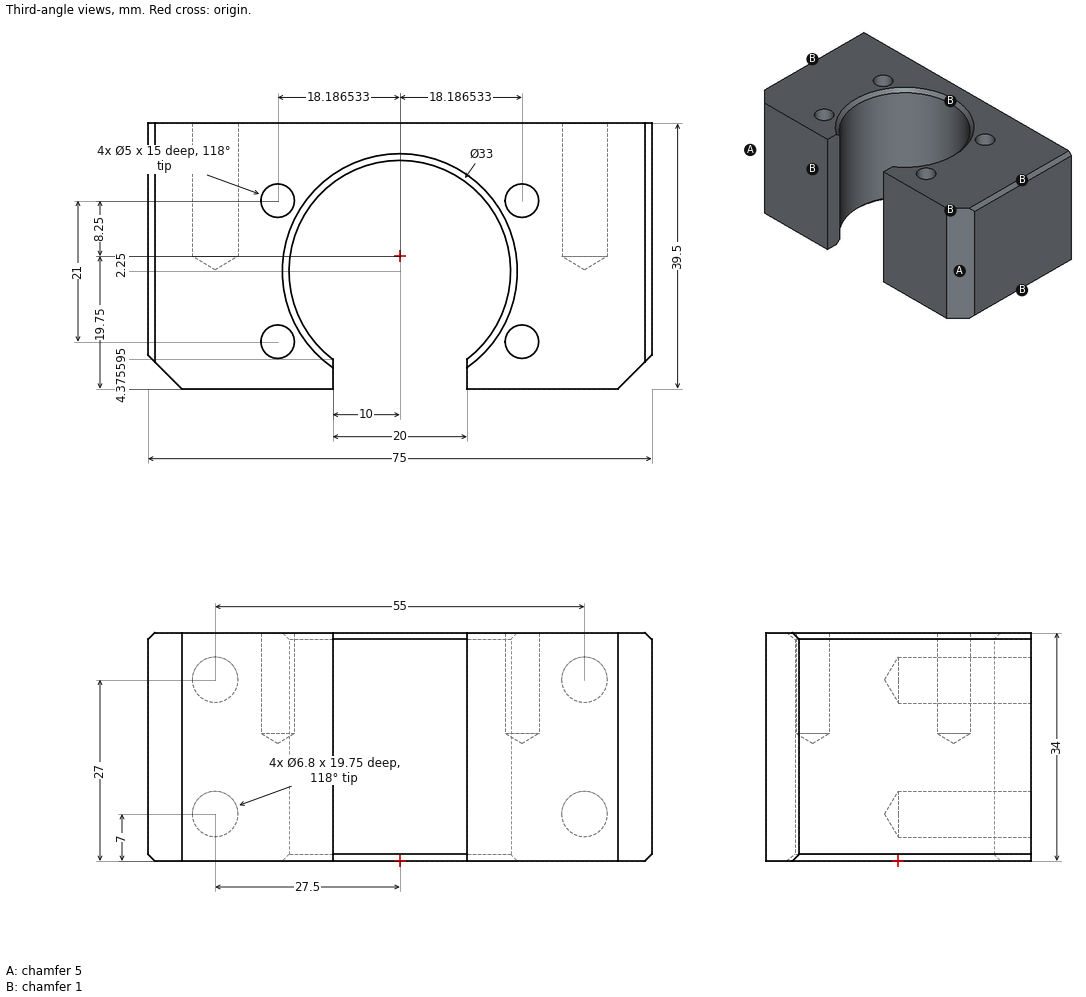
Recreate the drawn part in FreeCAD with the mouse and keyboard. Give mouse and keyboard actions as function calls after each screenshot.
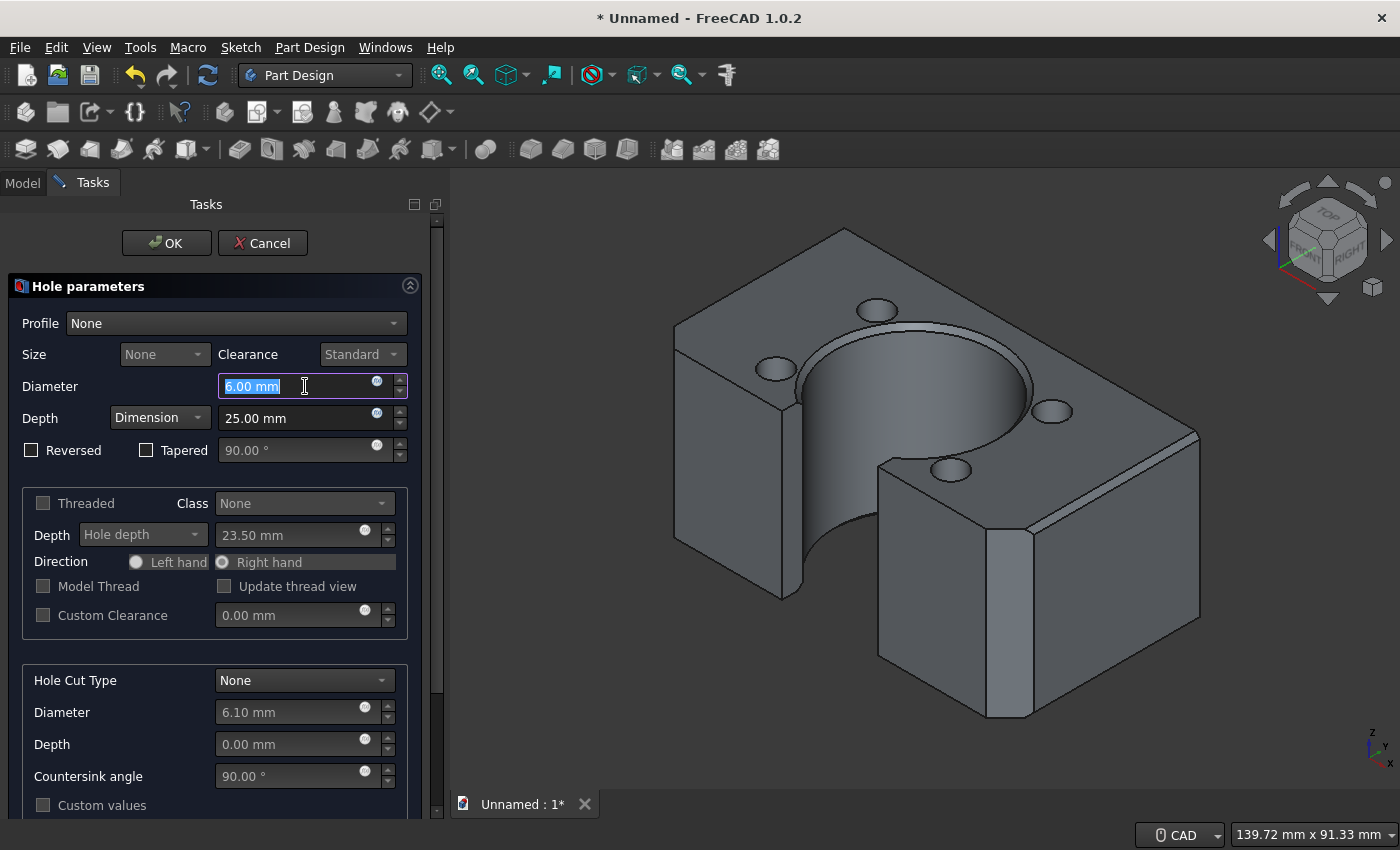
text(5)
key(Tab)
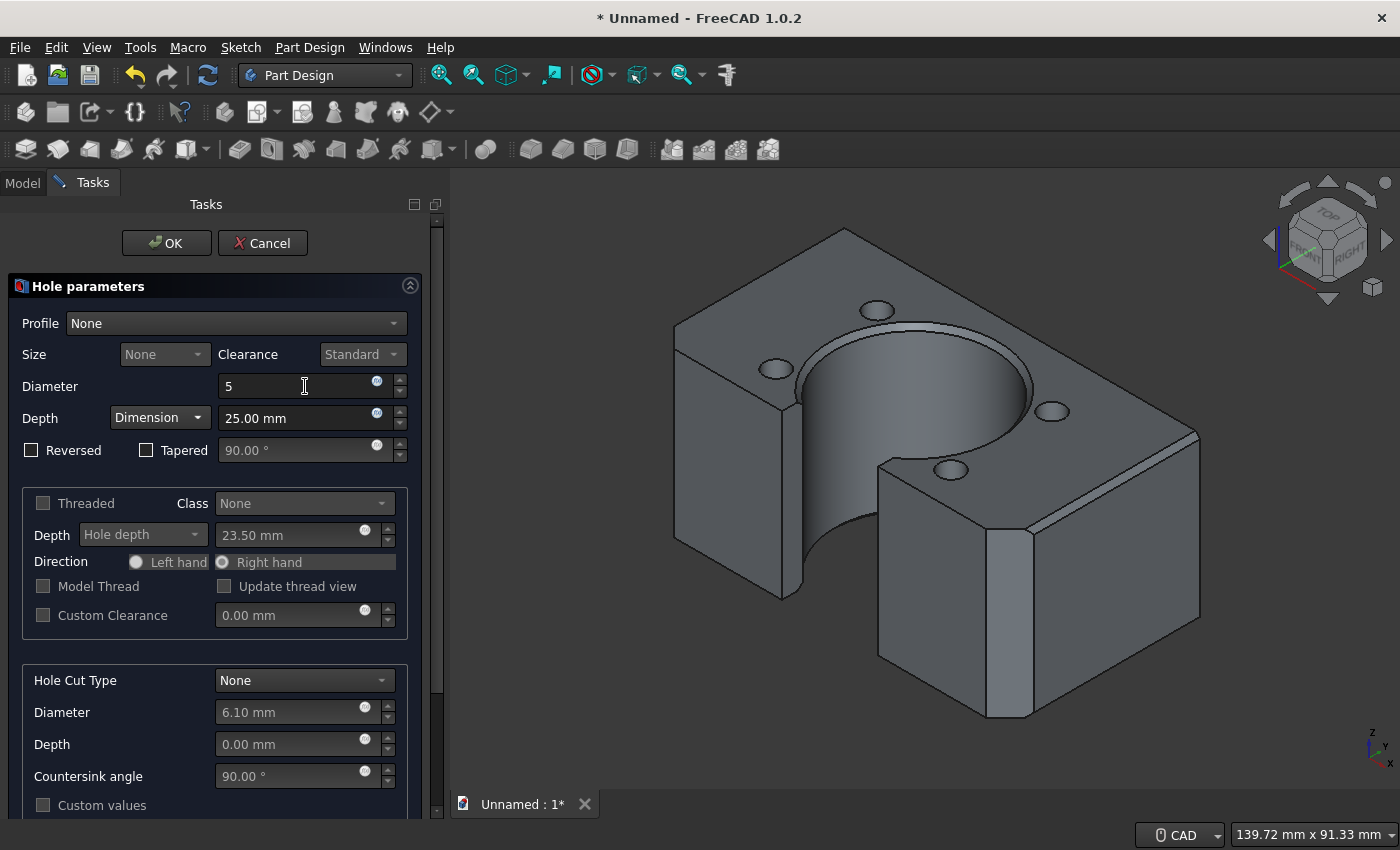
triple_click(305, 418)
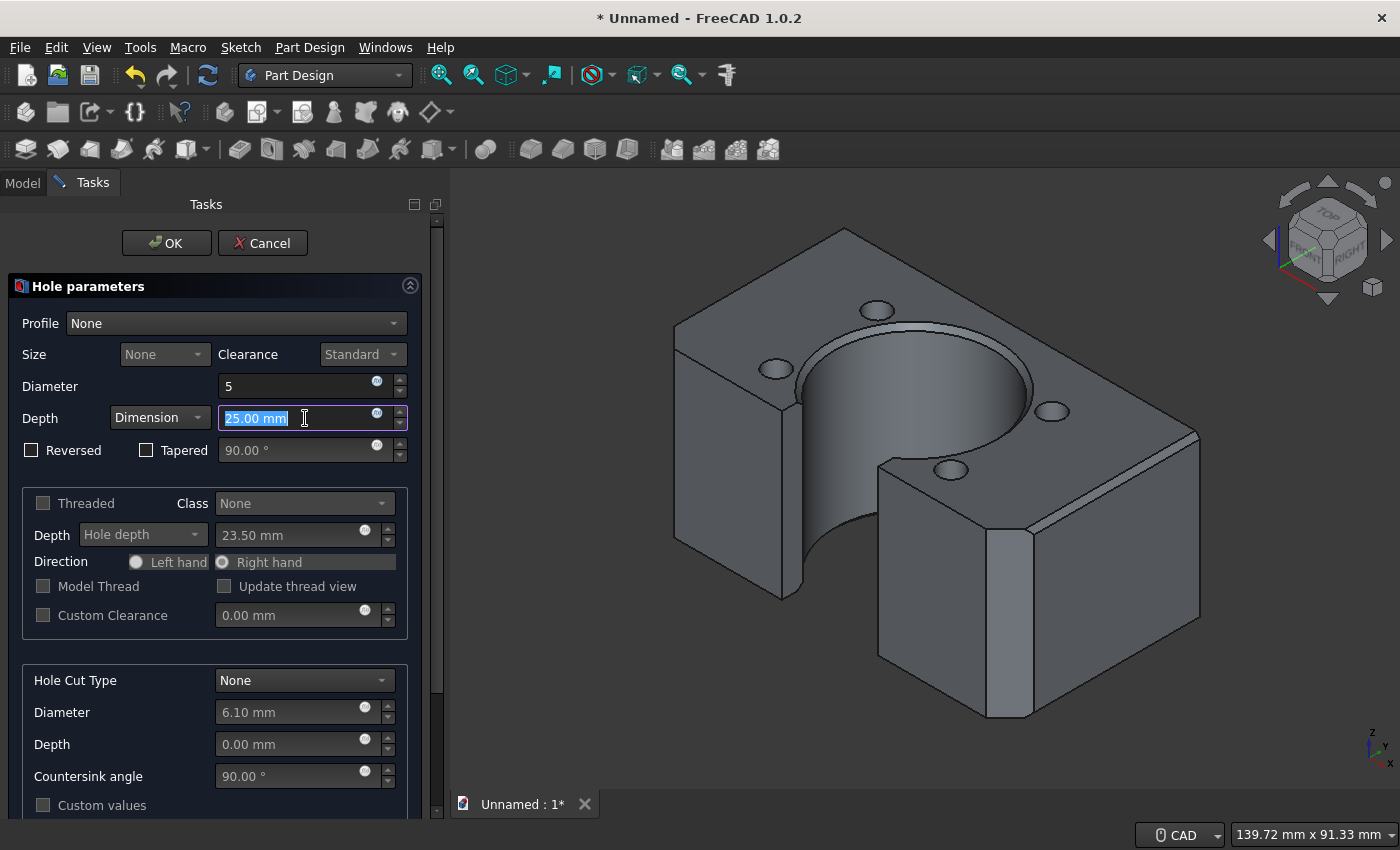
text(15)
key(Tab)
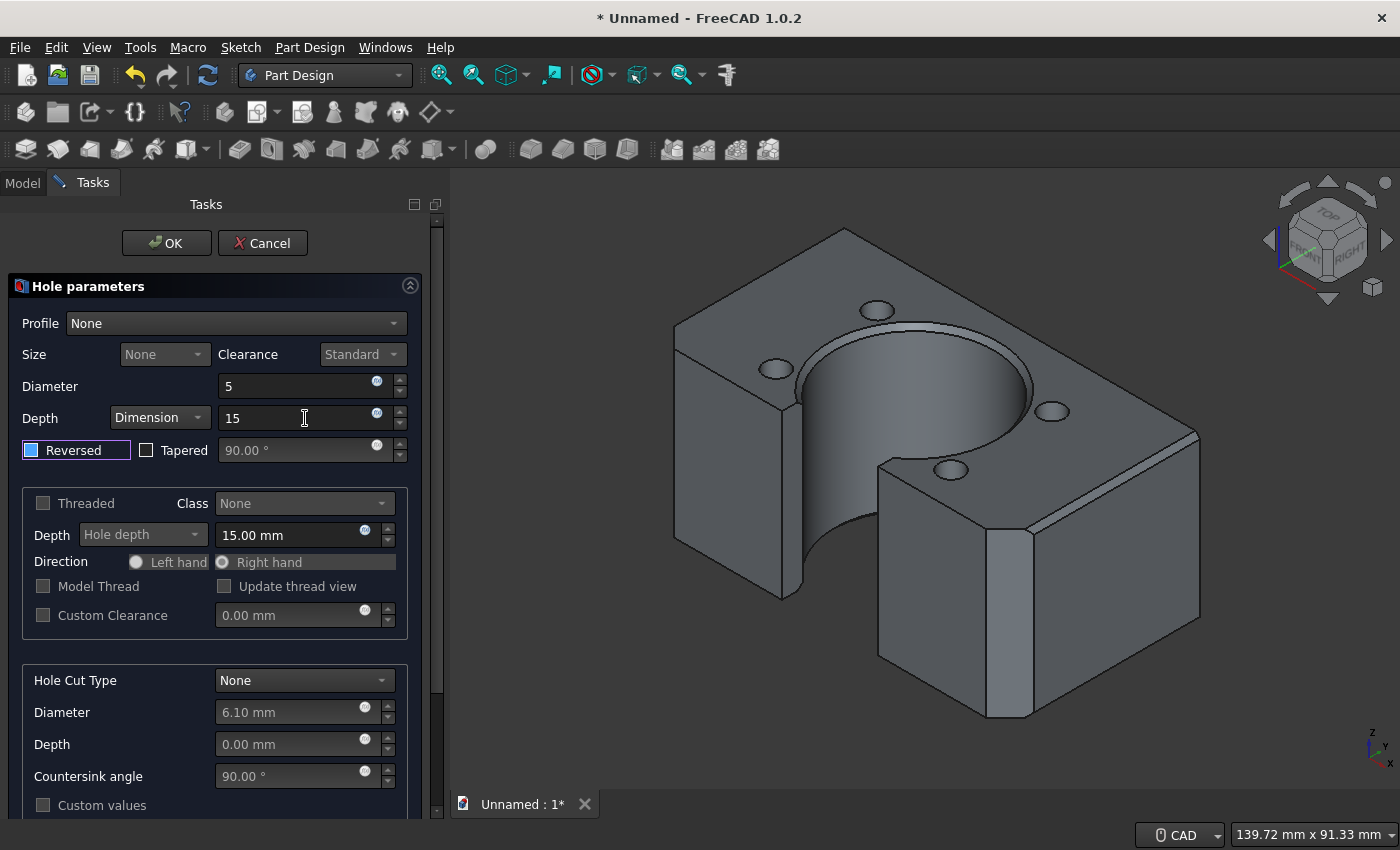
click(167, 243)